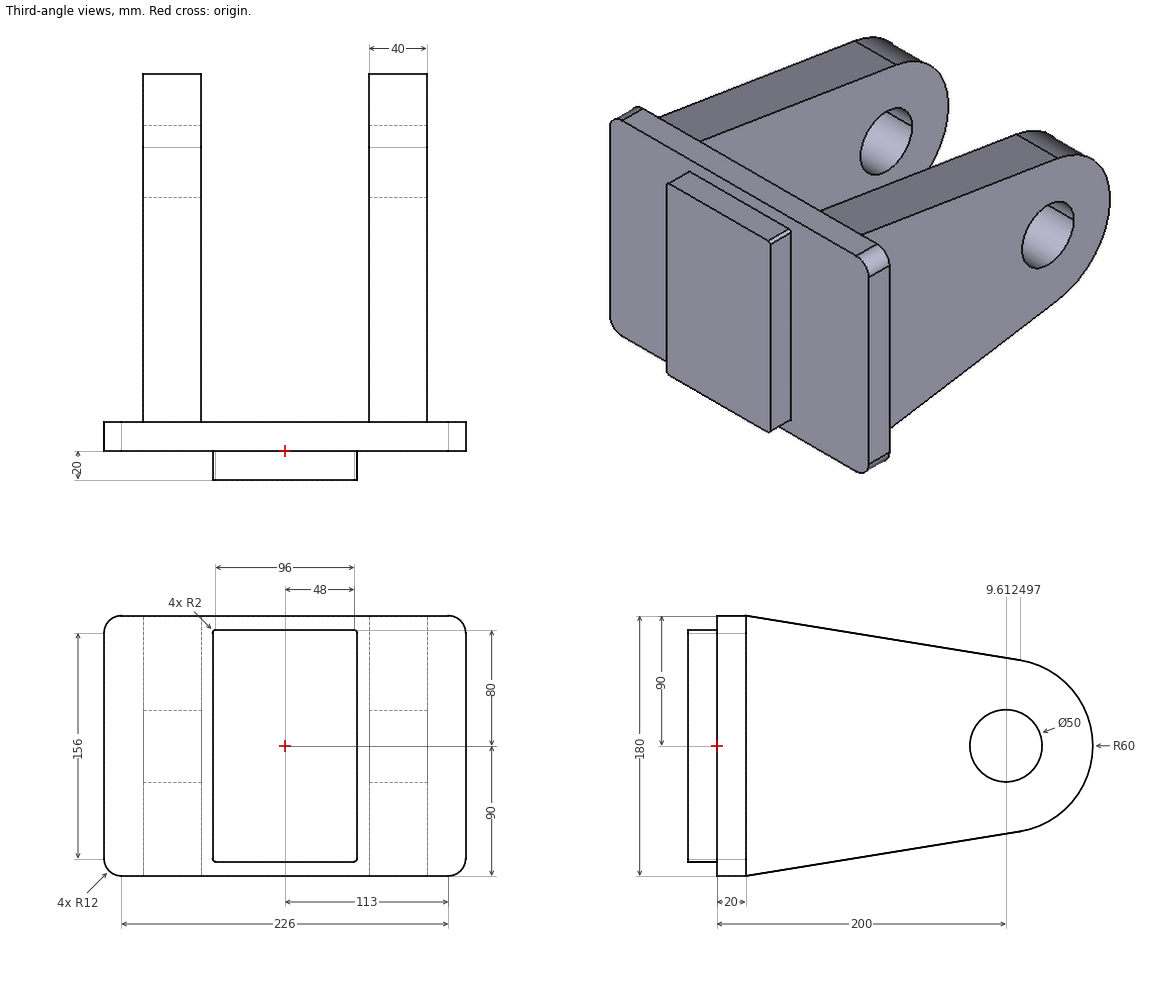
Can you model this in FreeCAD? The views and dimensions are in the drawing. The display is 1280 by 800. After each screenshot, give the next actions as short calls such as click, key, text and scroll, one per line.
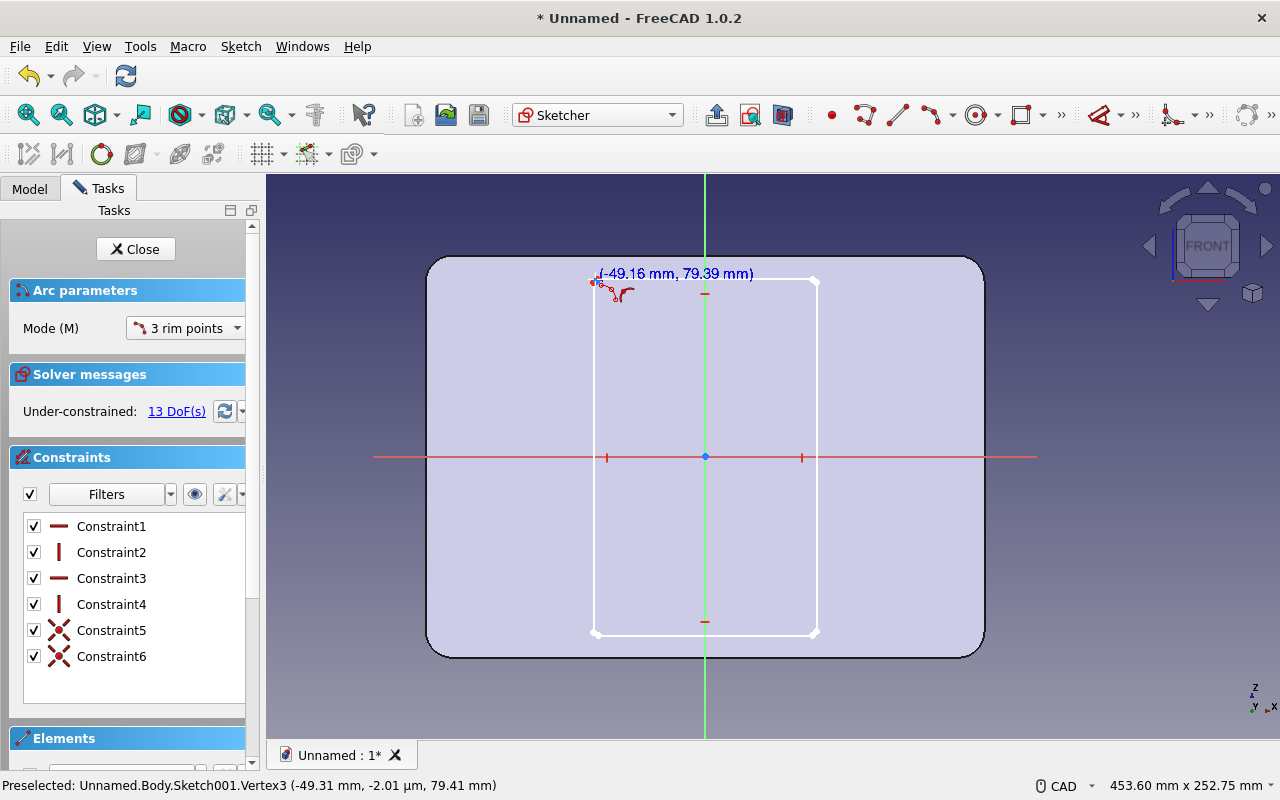
scroll(593, 631, up, 5)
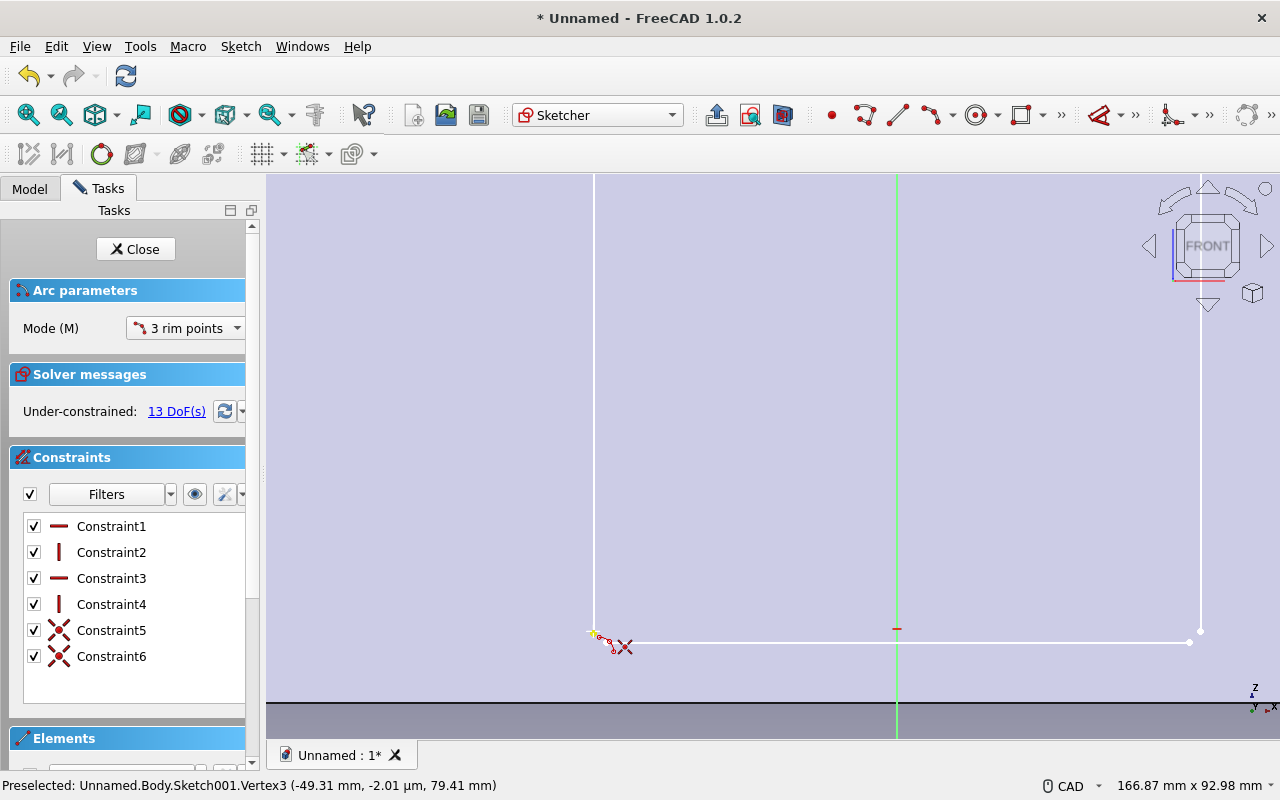
click(594, 633)
click(606, 643)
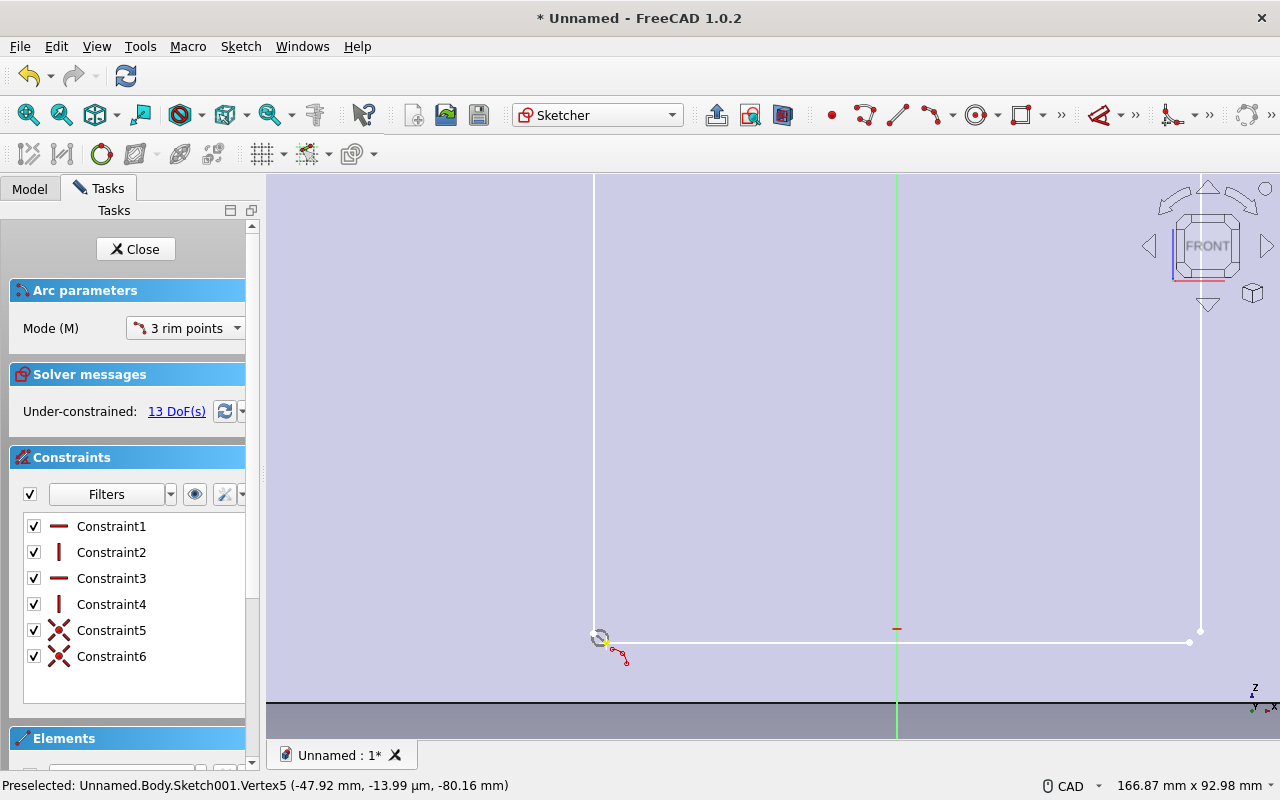
scroll(597, 638, up, 8)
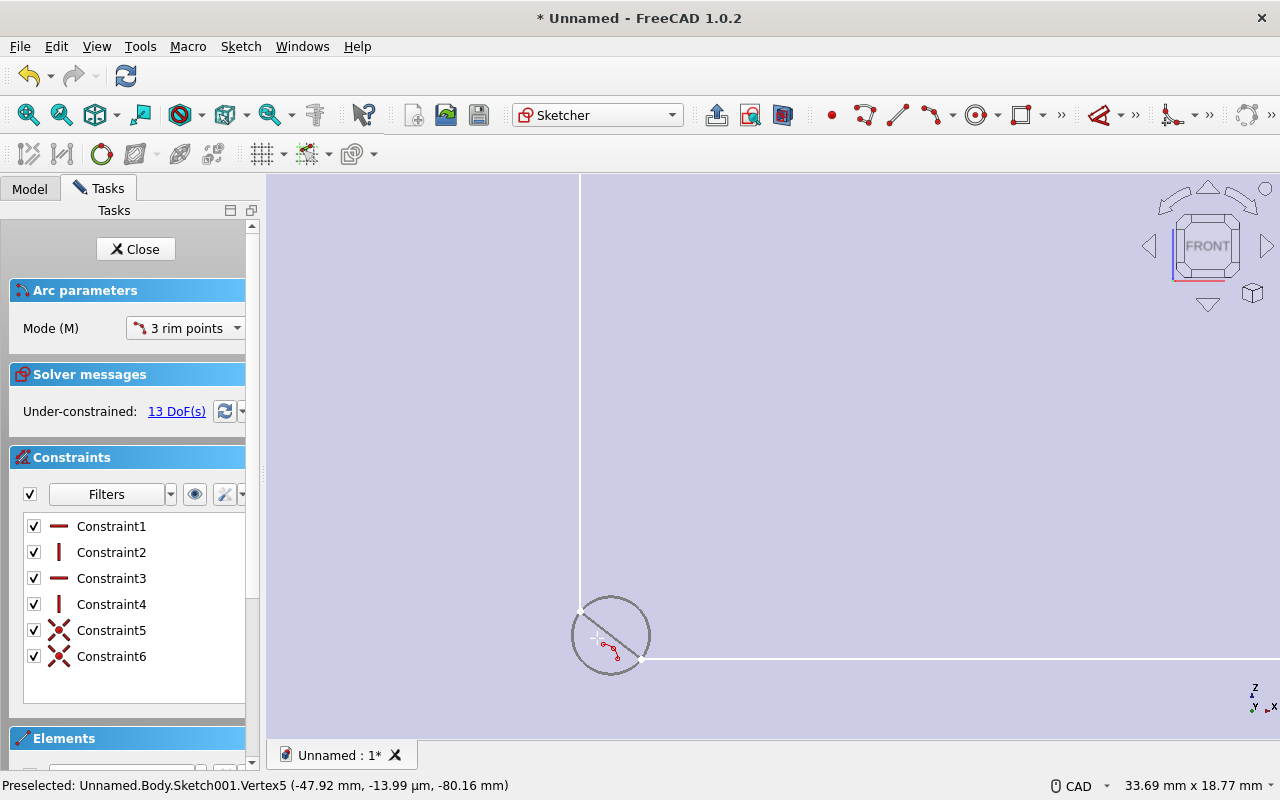
click(596, 637)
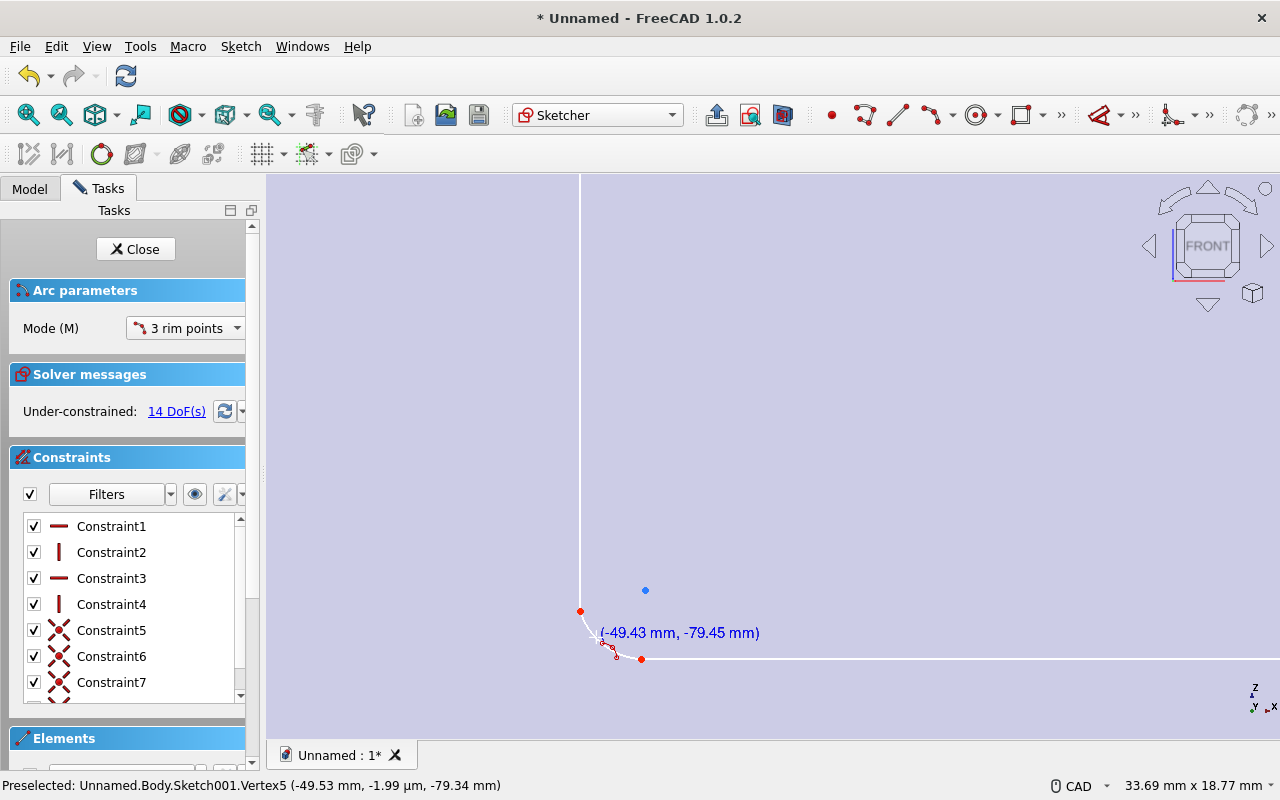
scroll(594, 634, down, 13)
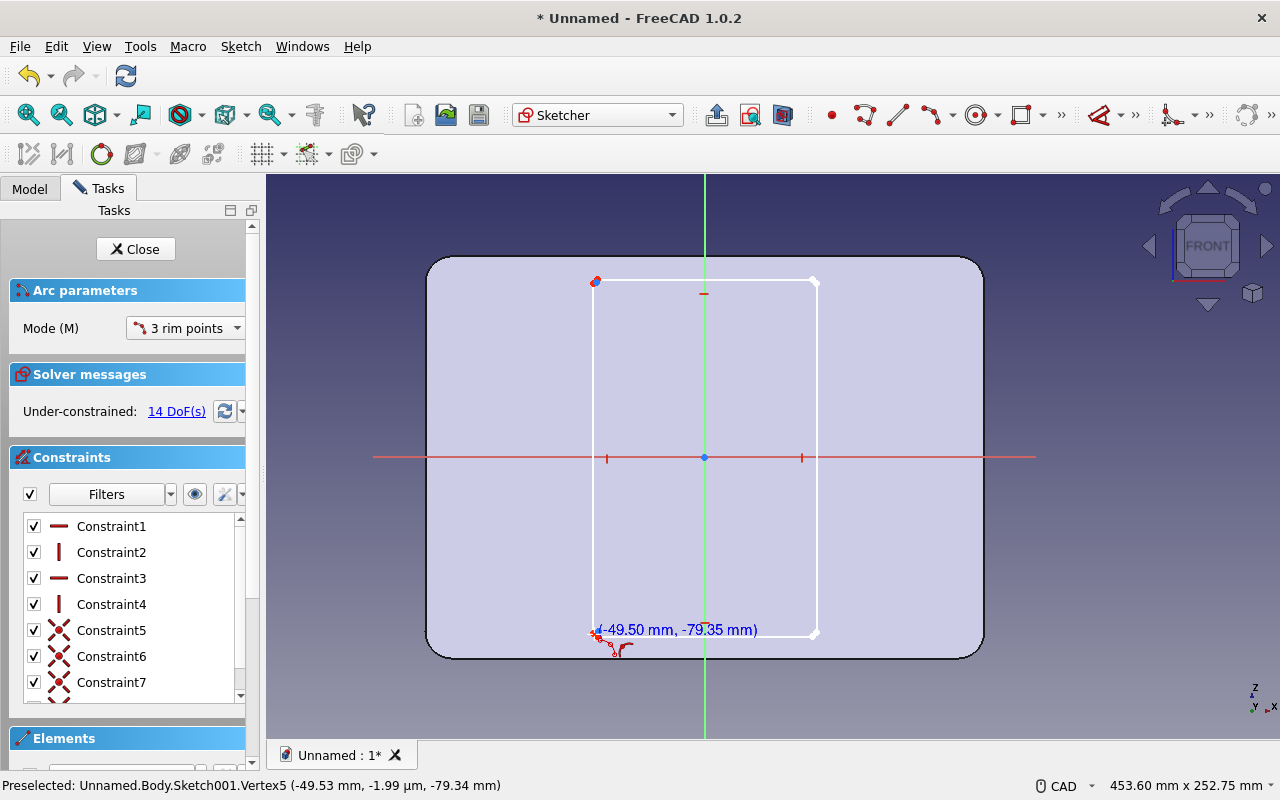
scroll(812, 636, up, 5)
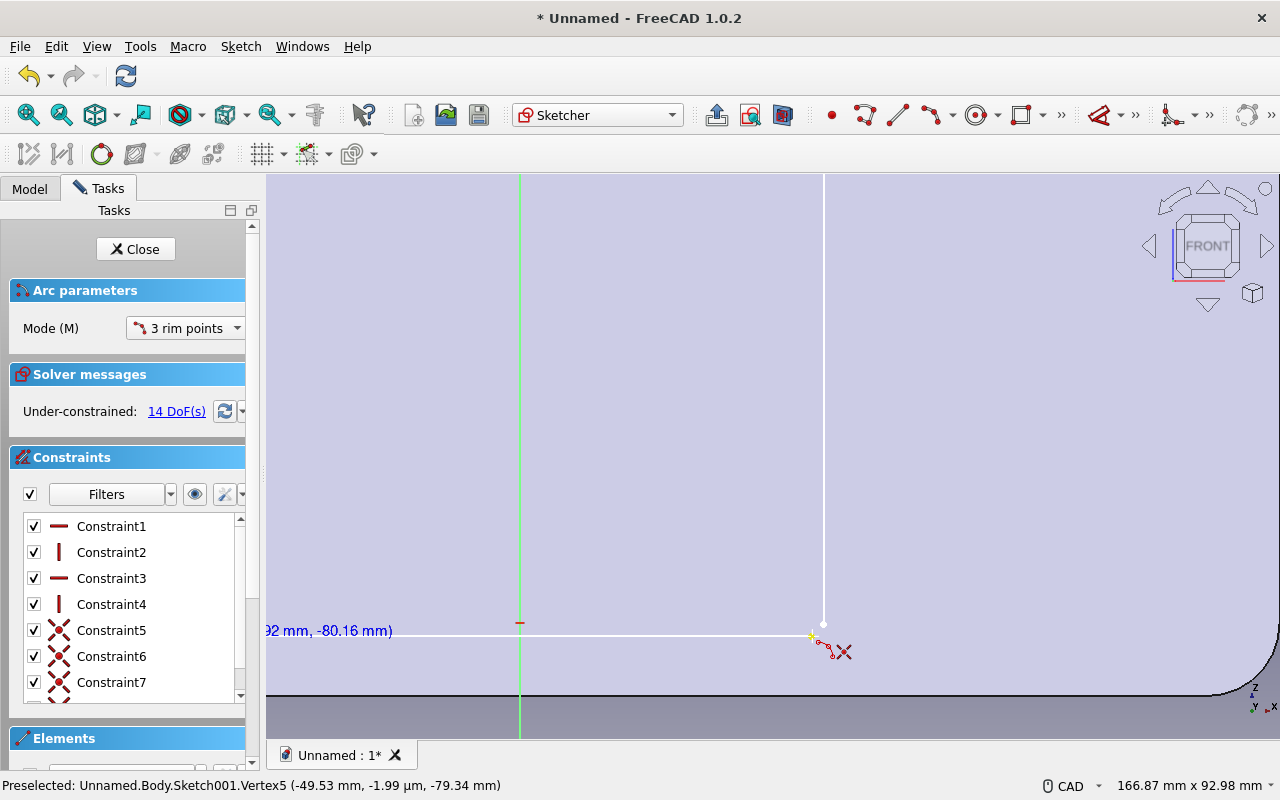
click(812, 636)
click(824, 625)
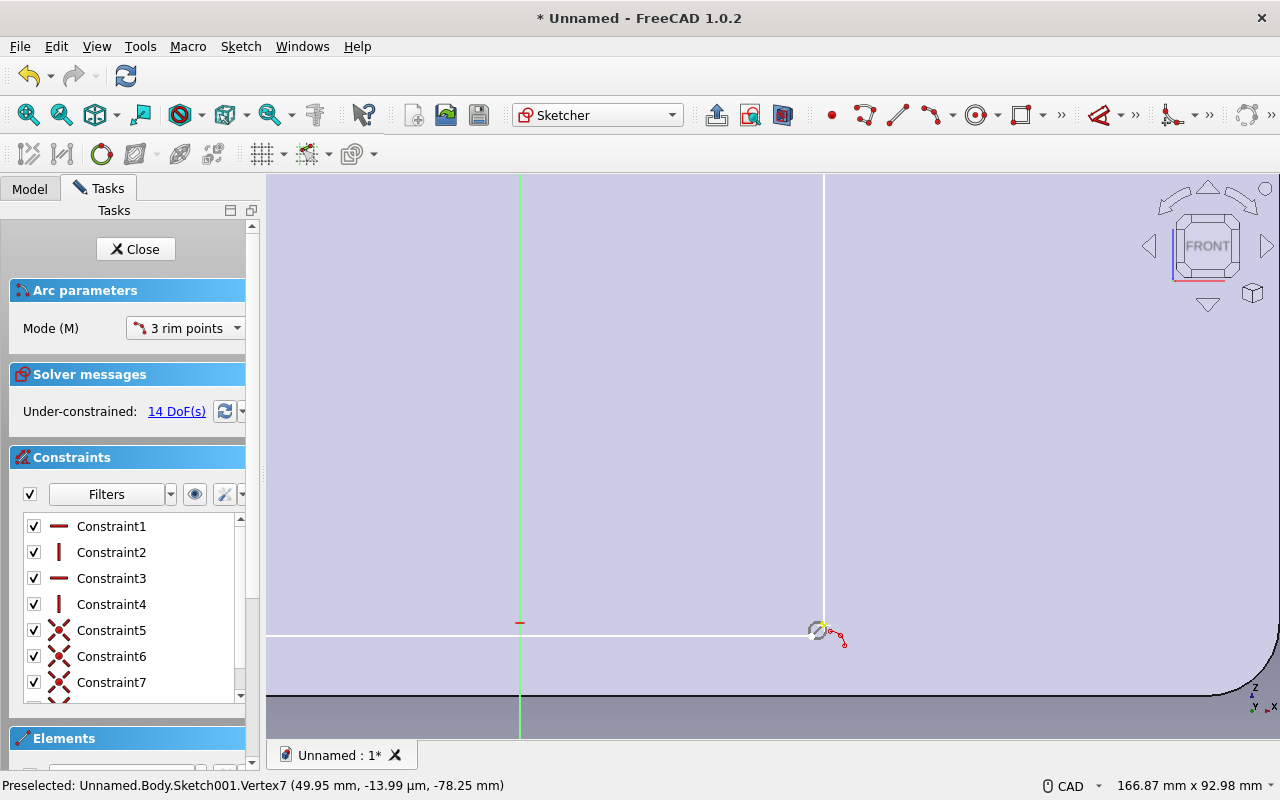
scroll(820, 632, up, 8)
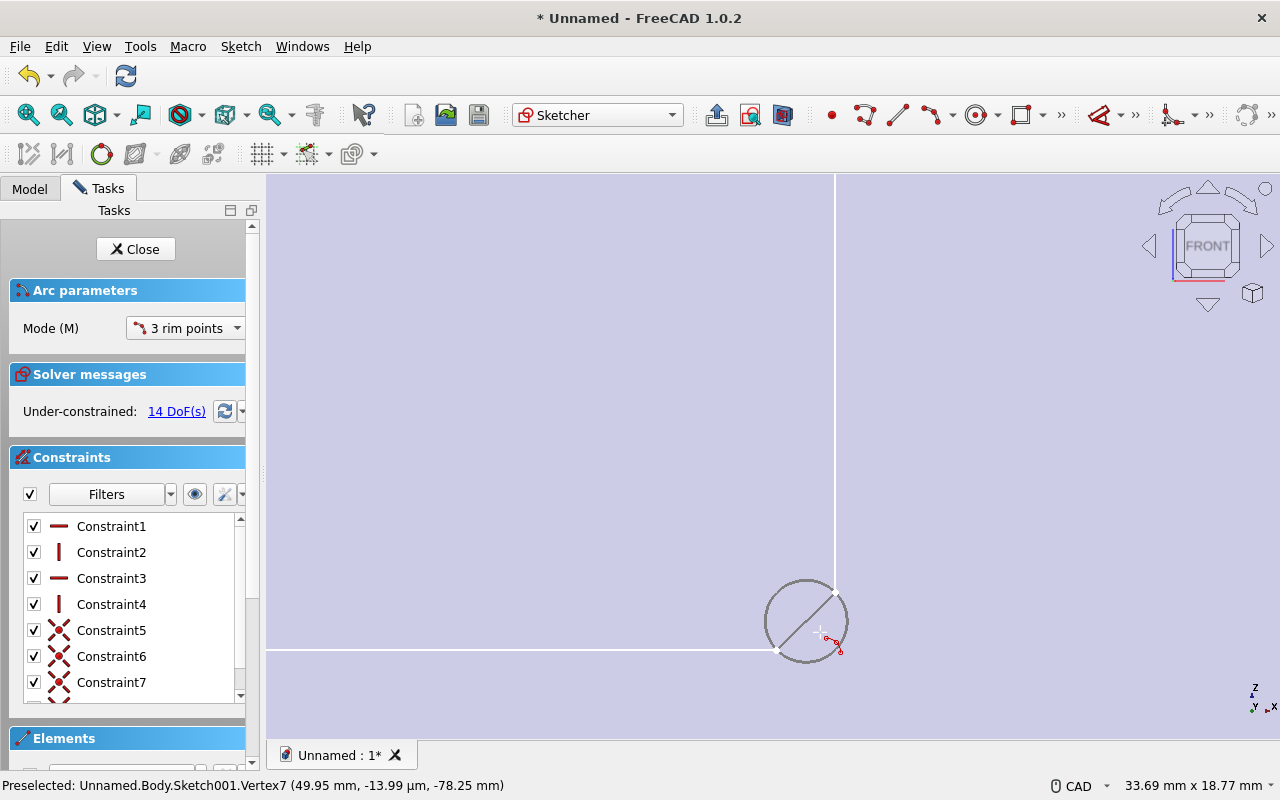
click(819, 628)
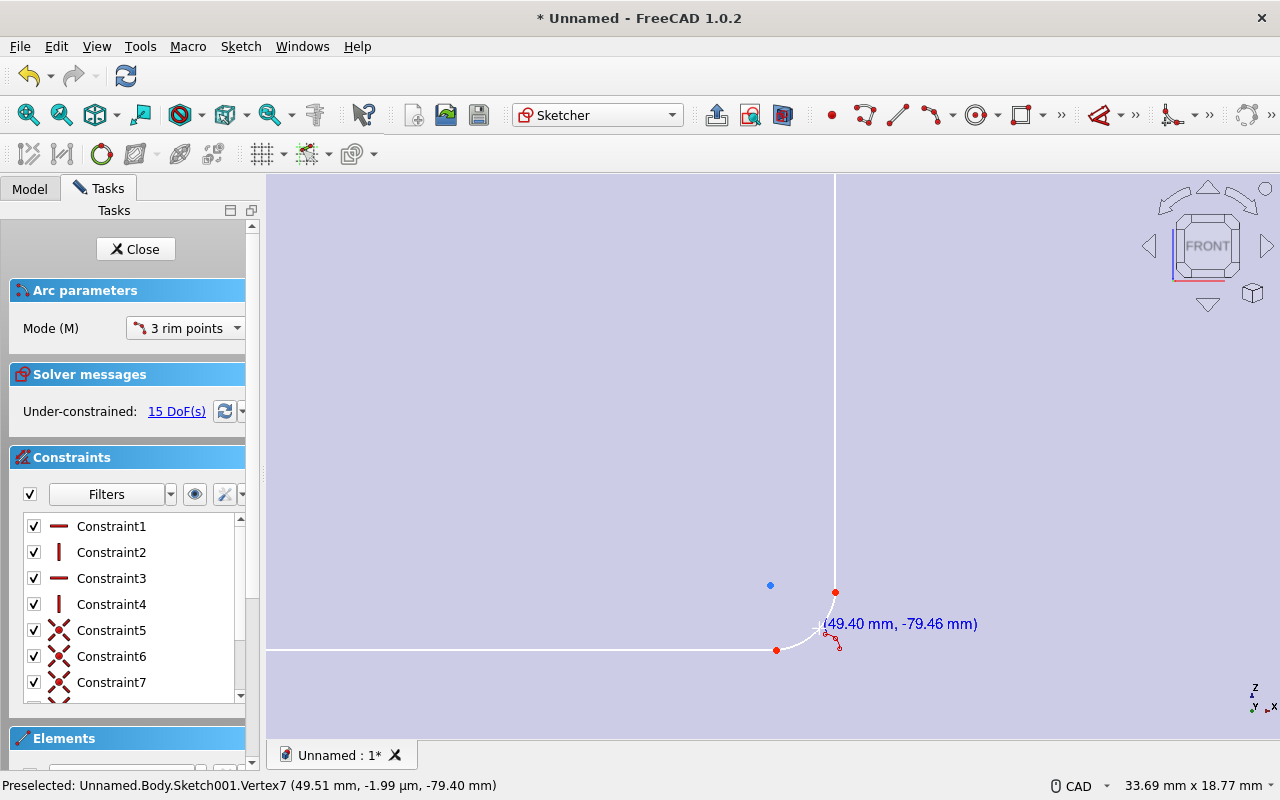
scroll(815, 635, down, 13)